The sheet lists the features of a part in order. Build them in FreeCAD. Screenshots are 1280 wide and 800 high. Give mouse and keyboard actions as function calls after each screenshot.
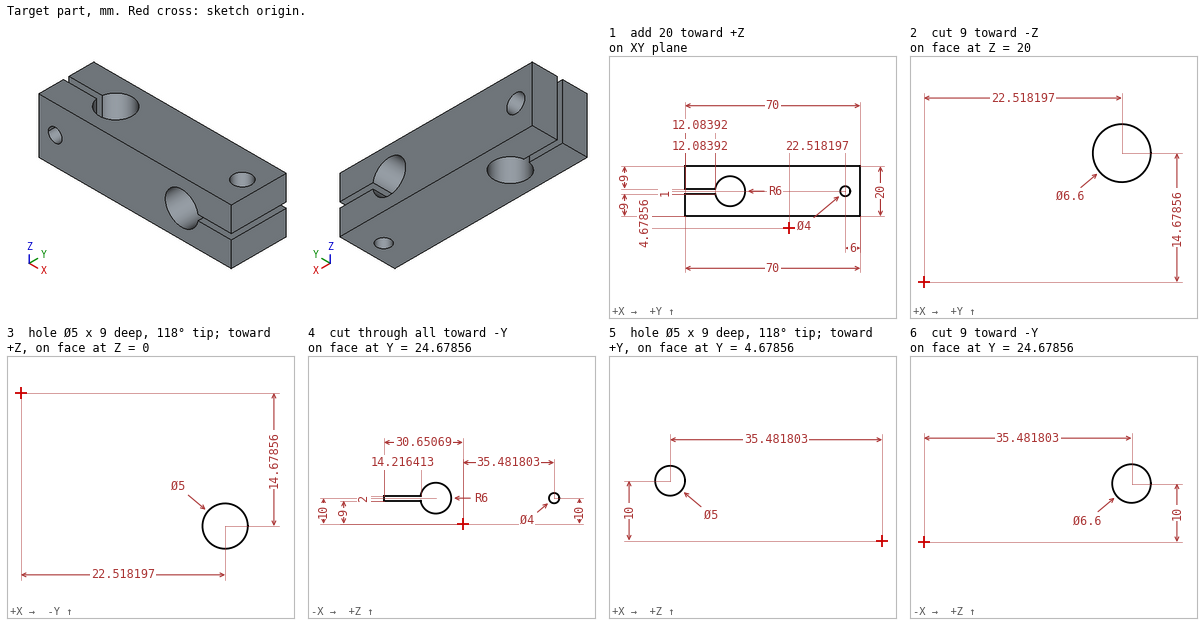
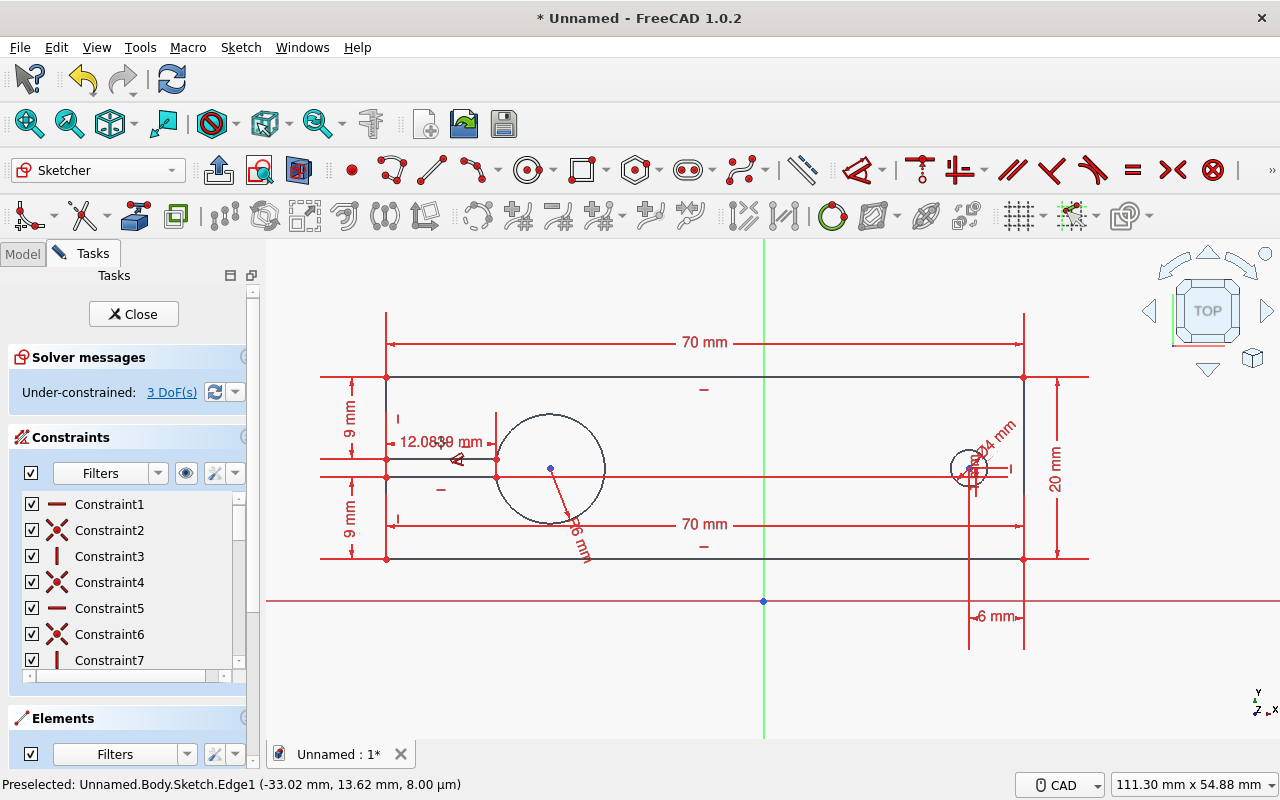
click(419, 459)
click(441, 493)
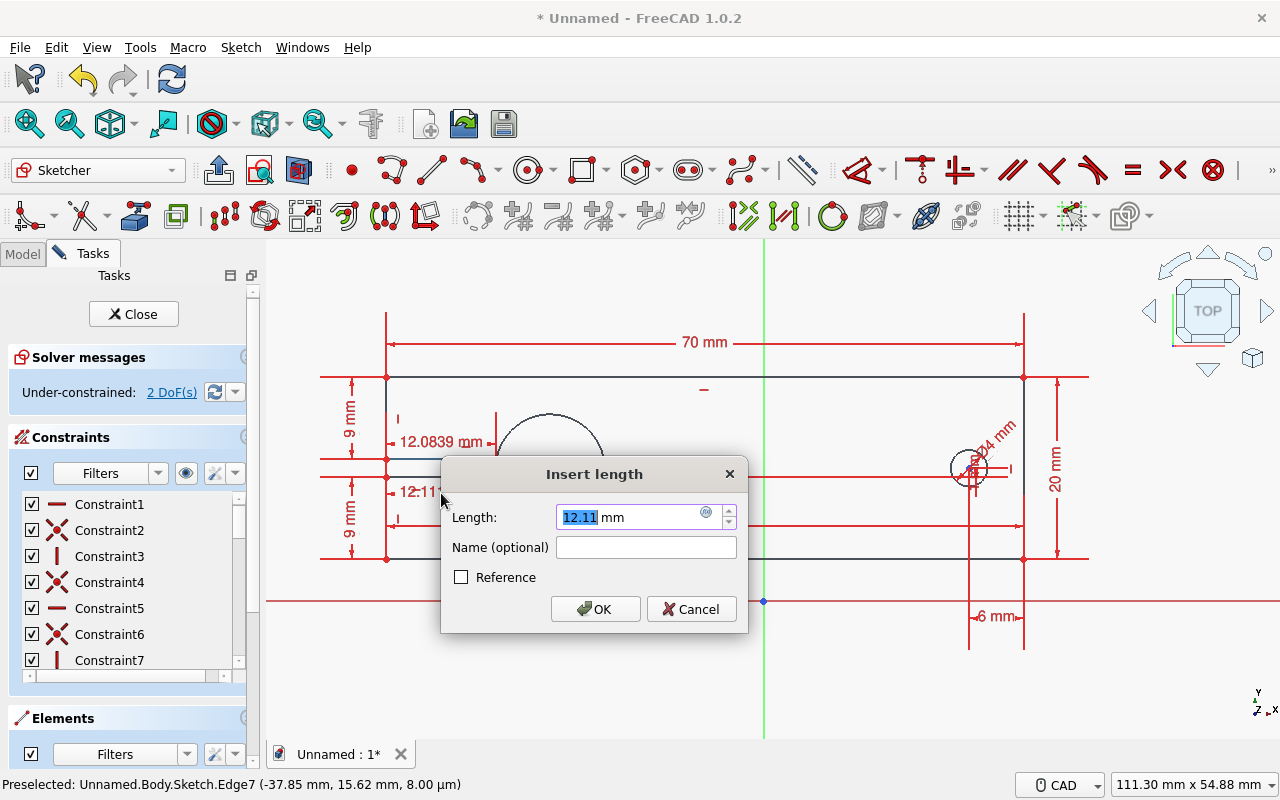
text(12.08392)
key(Return)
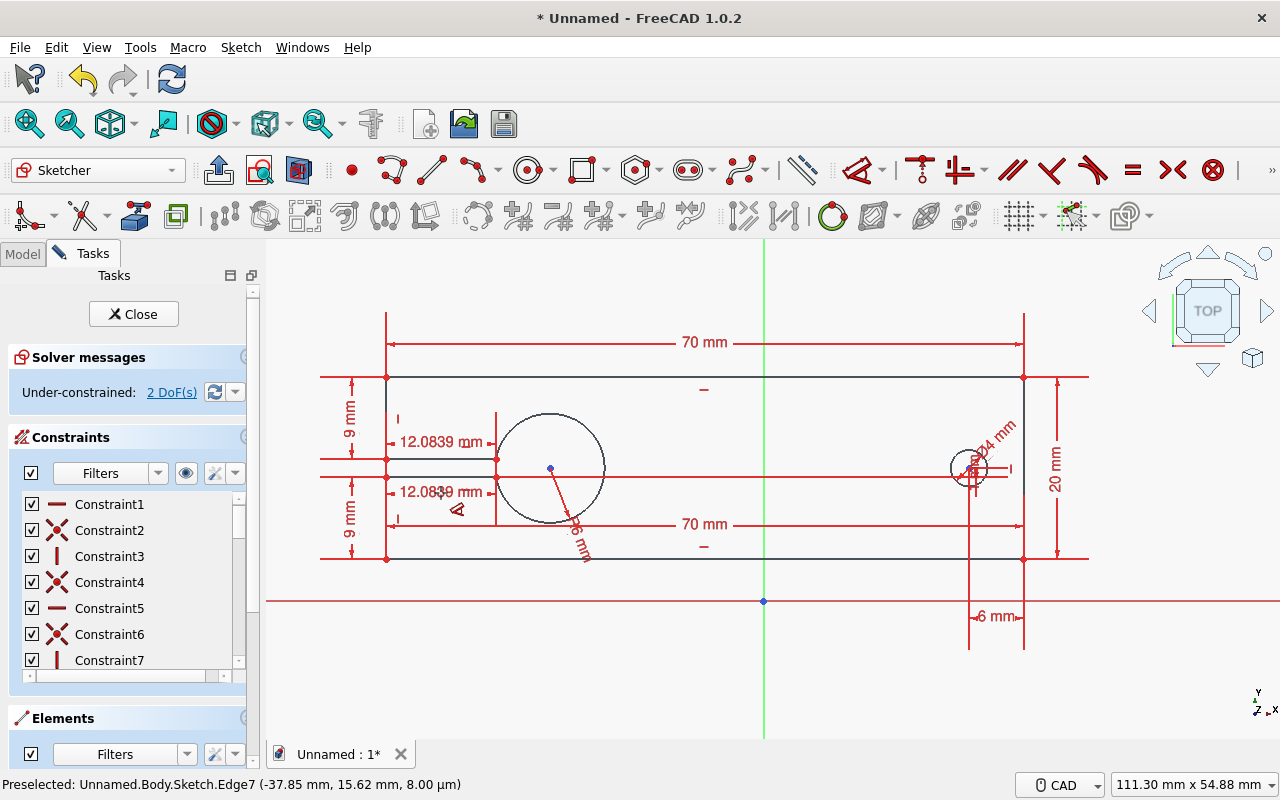
click(386, 559)
click(352, 580)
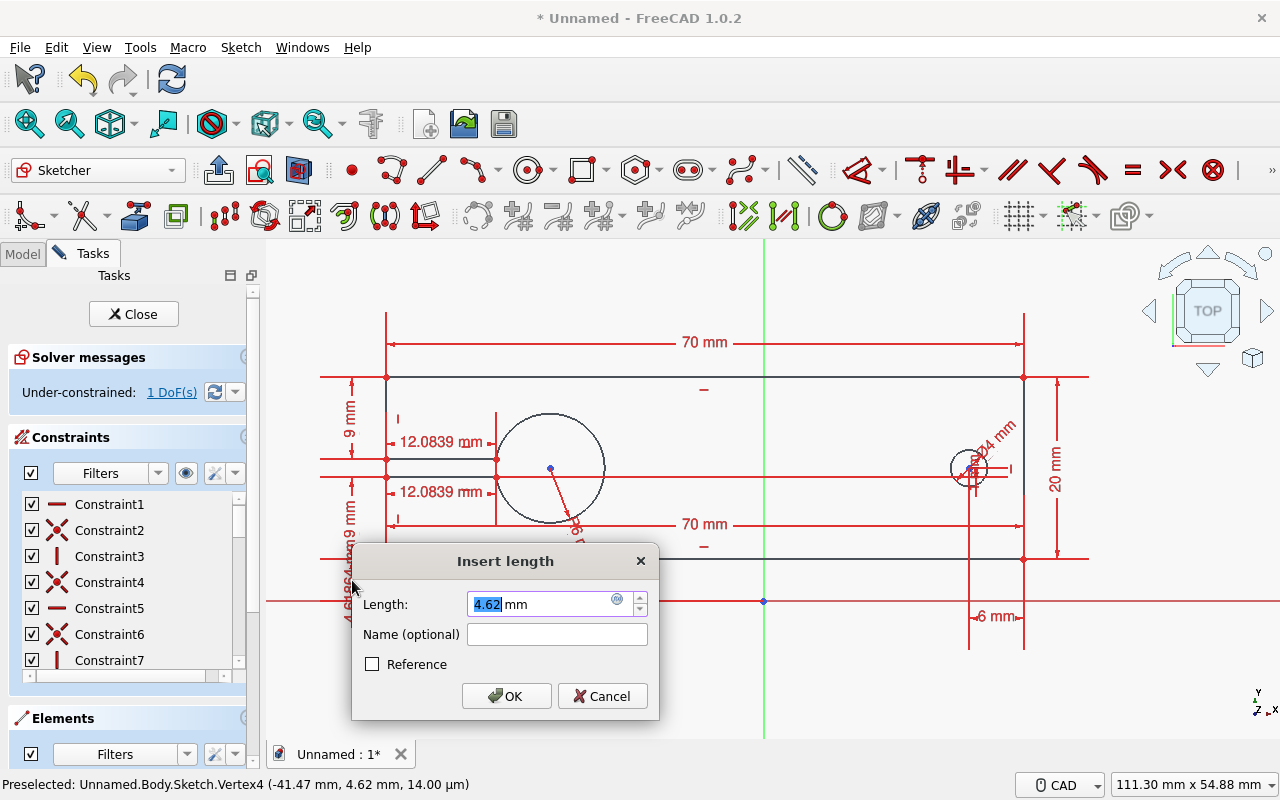
text(4.67856)
key(Return)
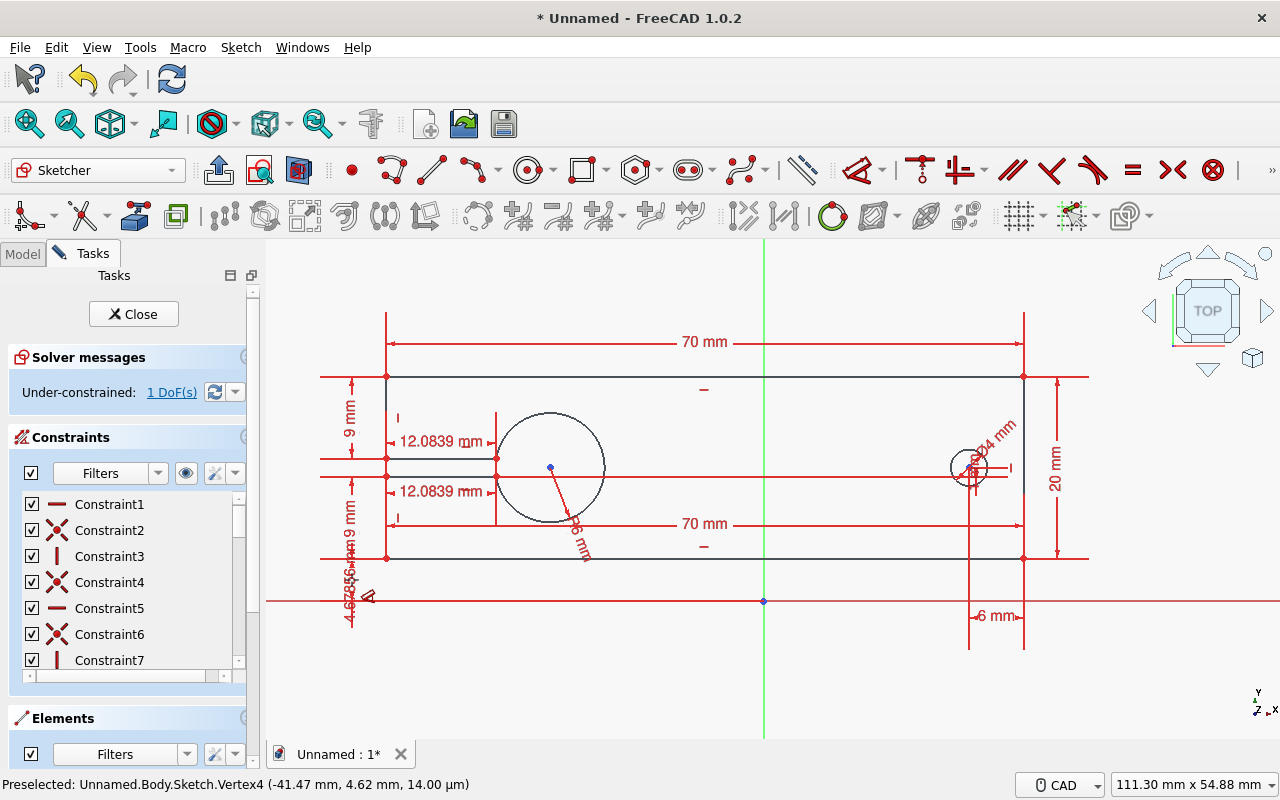
click(969, 468)
click(866, 635)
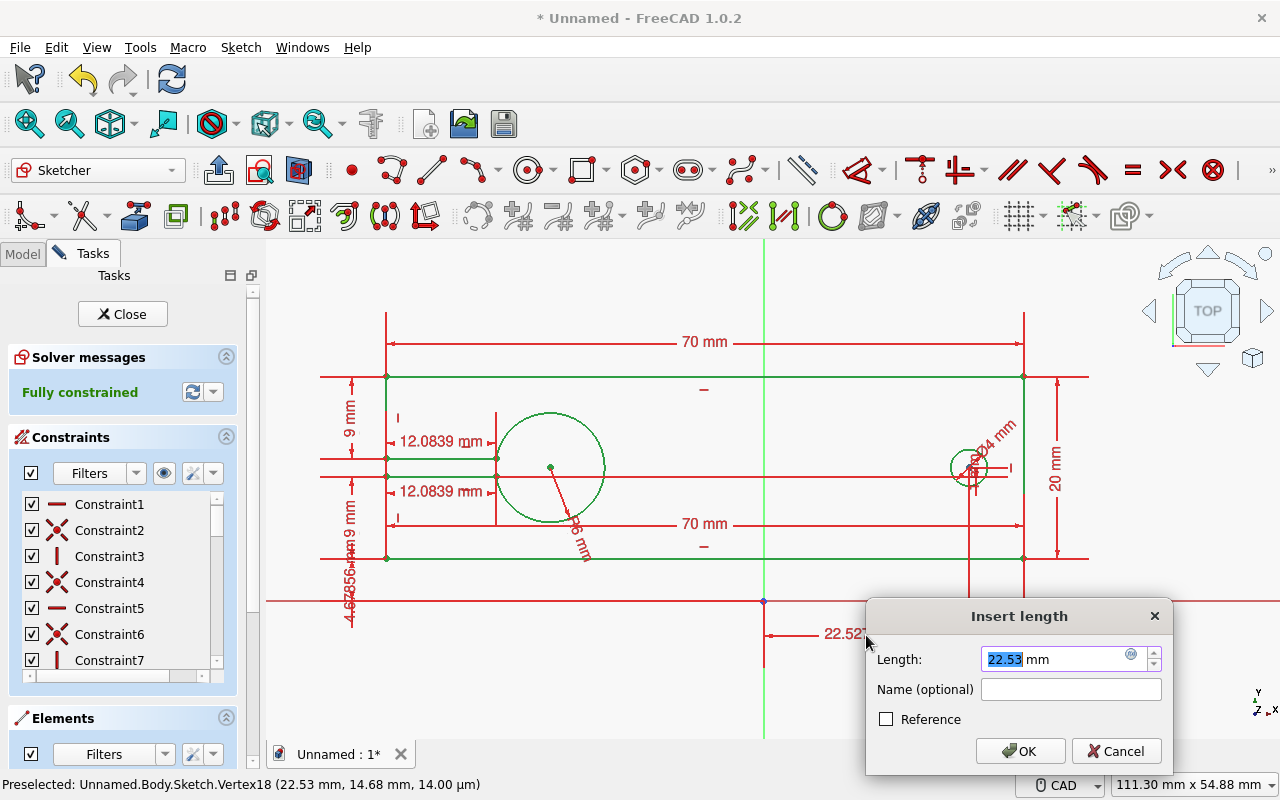
text(22.518197)
key(Return)
key(Escape)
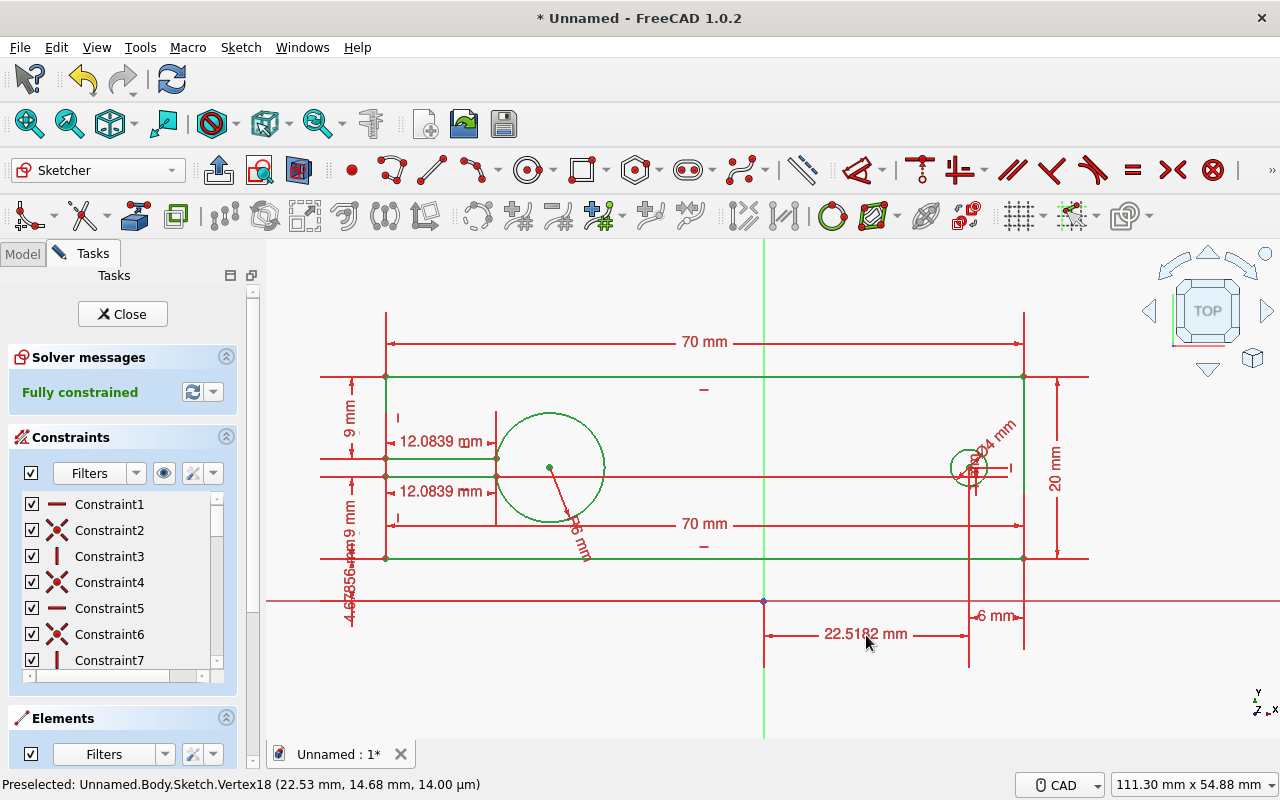
click(123, 314)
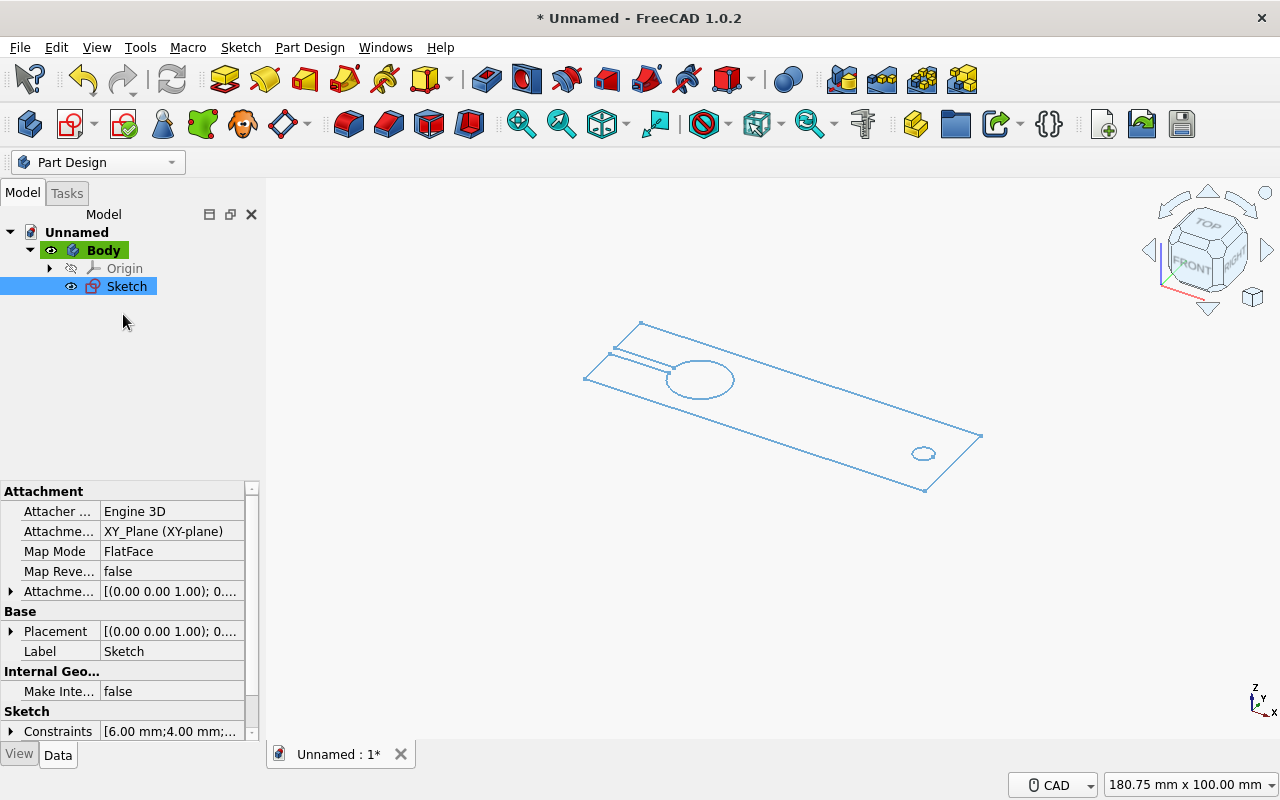
click(226, 80)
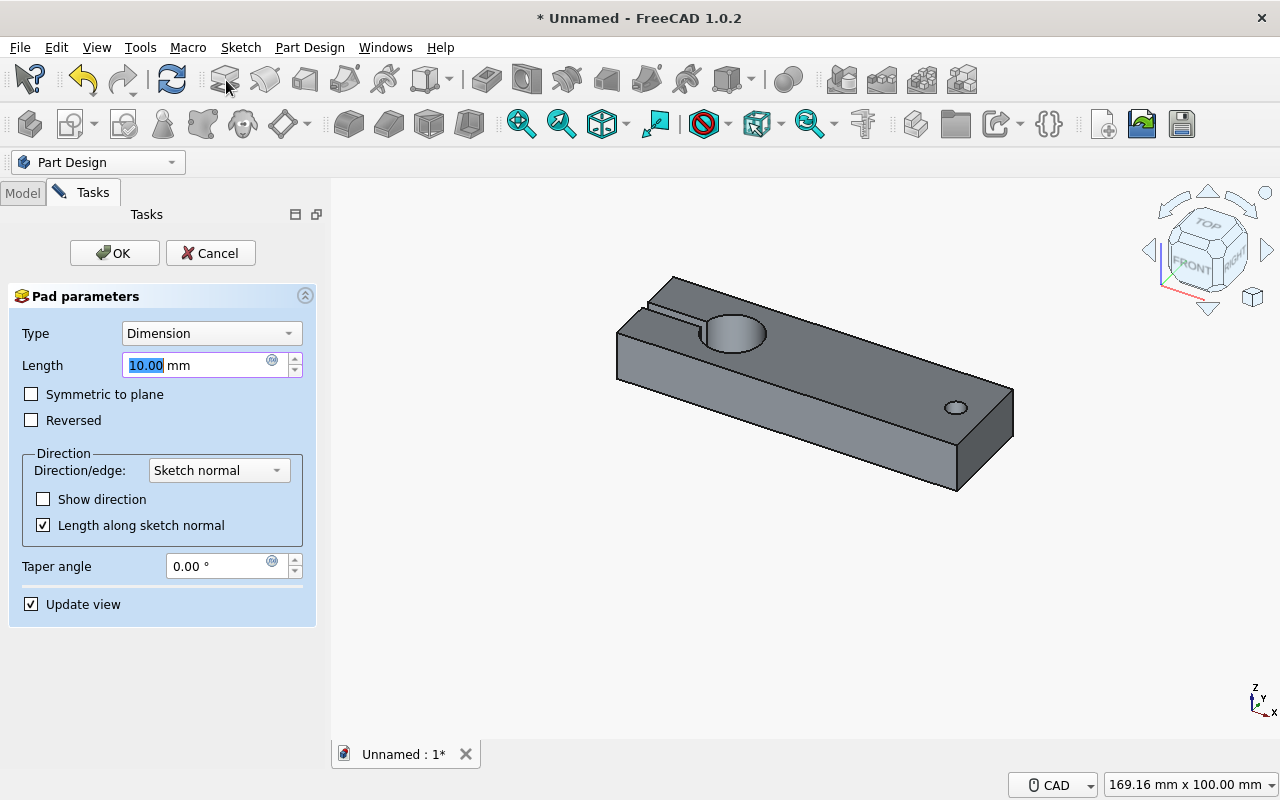
text(20)
key(Tab)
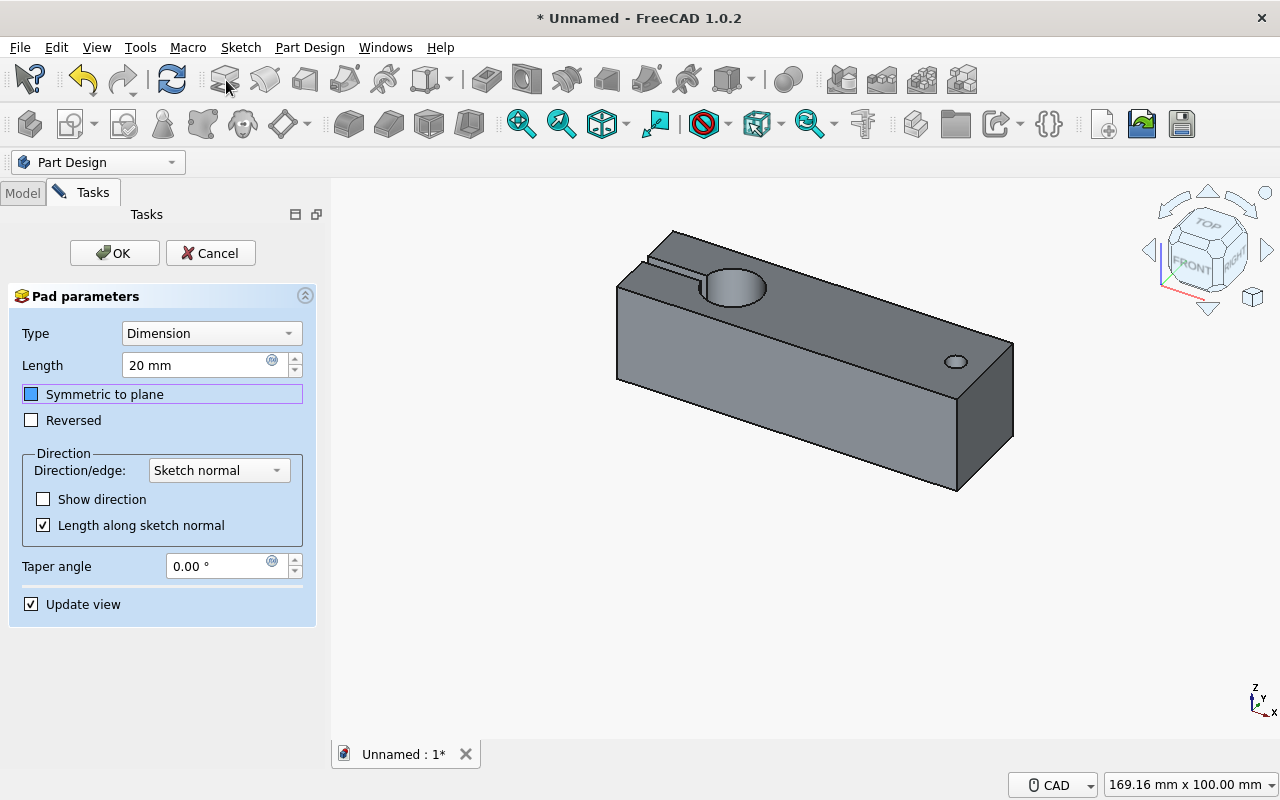
click(115, 253)